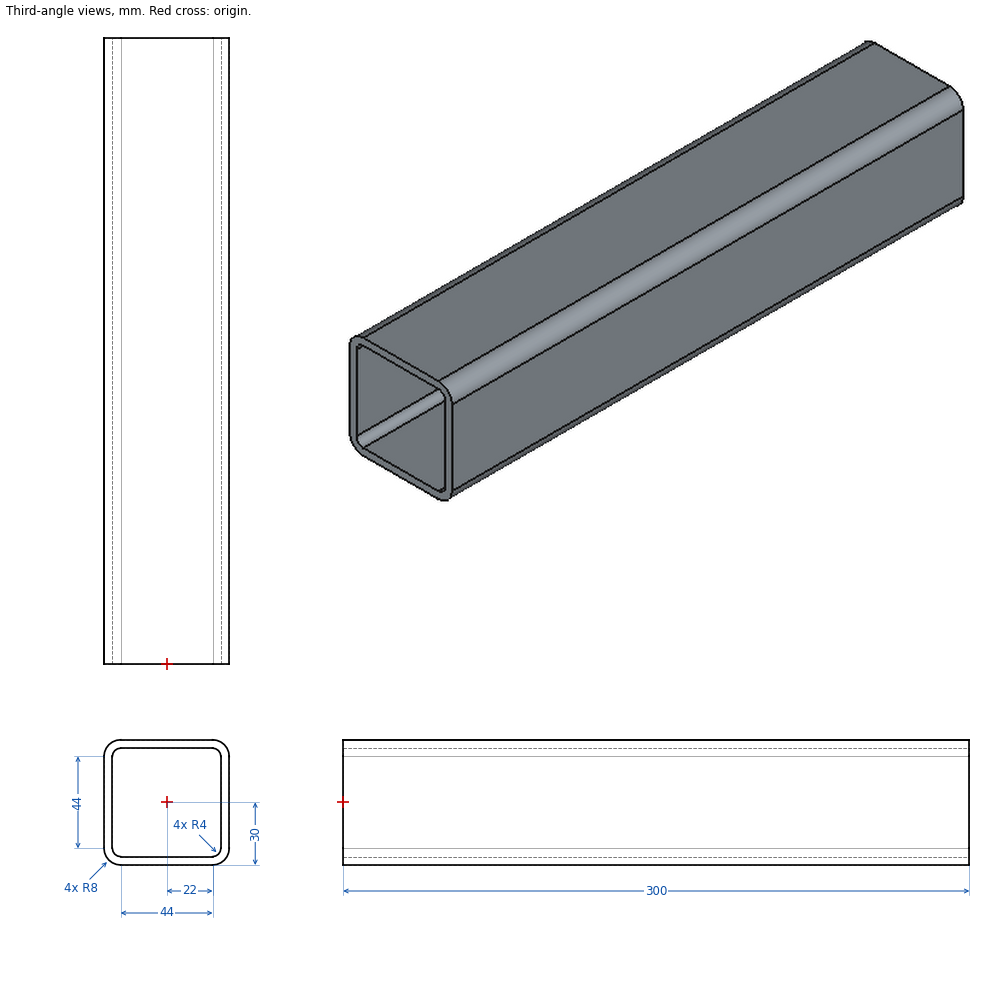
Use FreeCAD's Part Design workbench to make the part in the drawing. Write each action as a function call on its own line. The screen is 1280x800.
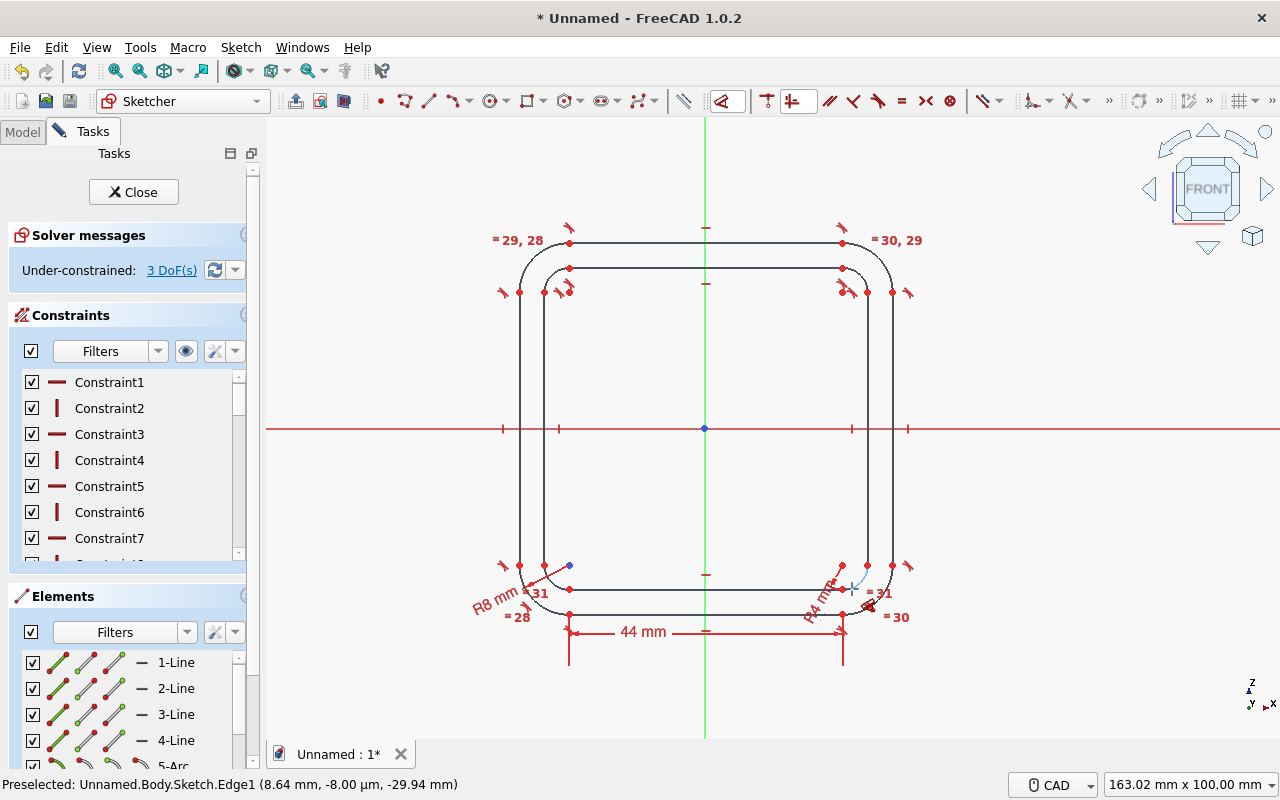
click(520, 483)
click(486, 366)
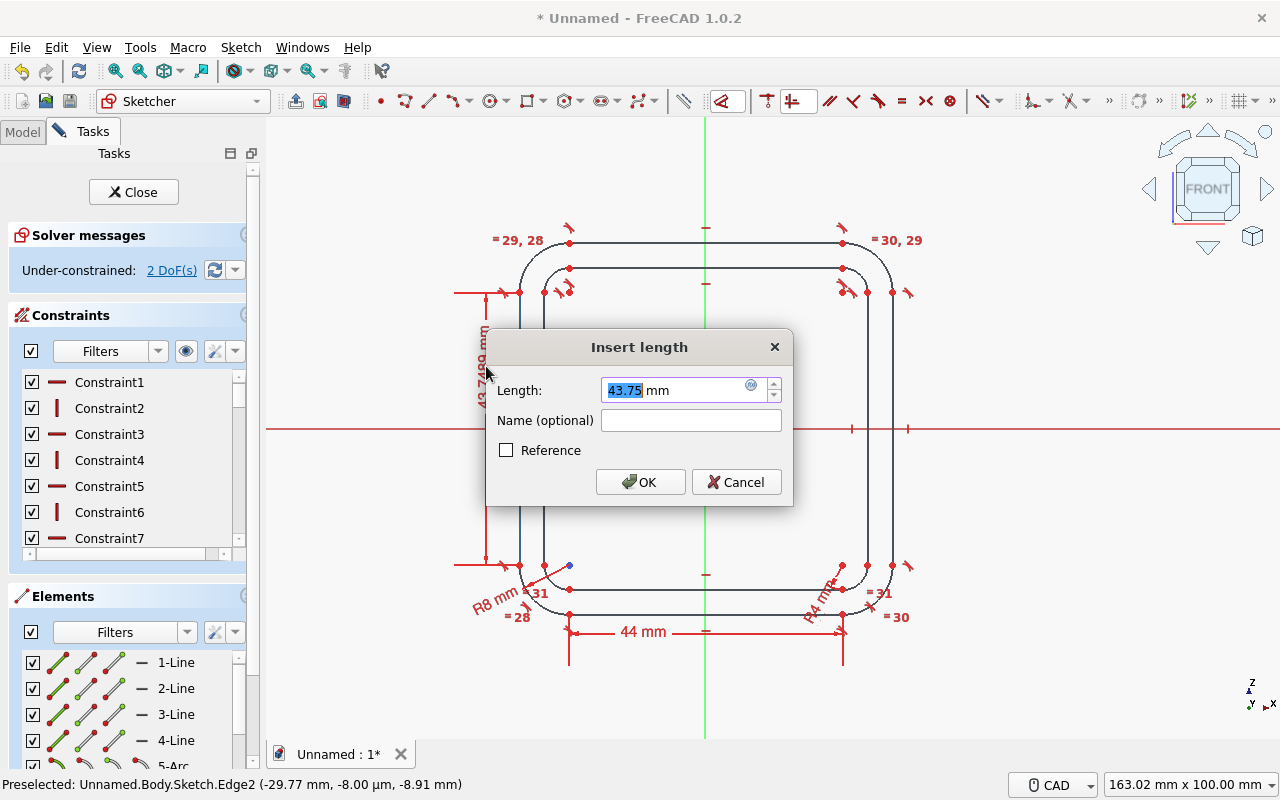
text(44)
key(Return)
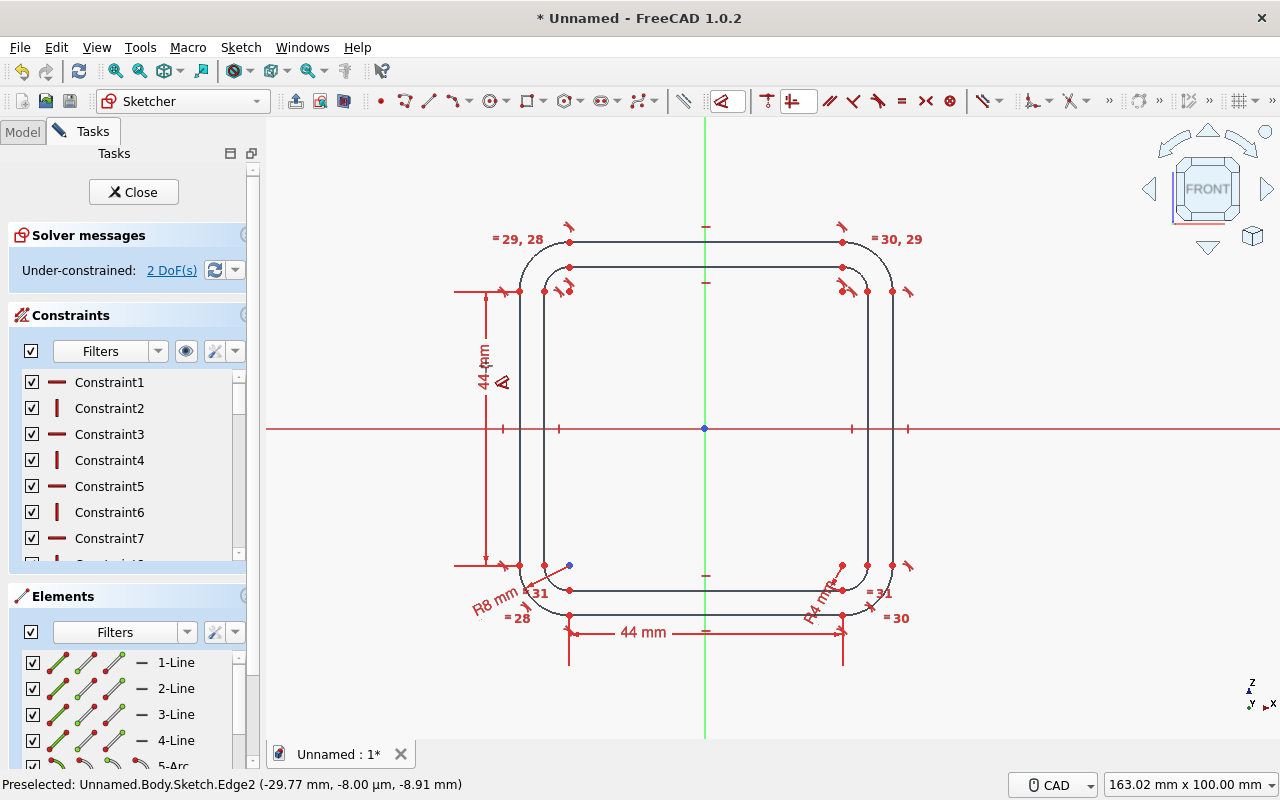
click(843, 615)
click(774, 649)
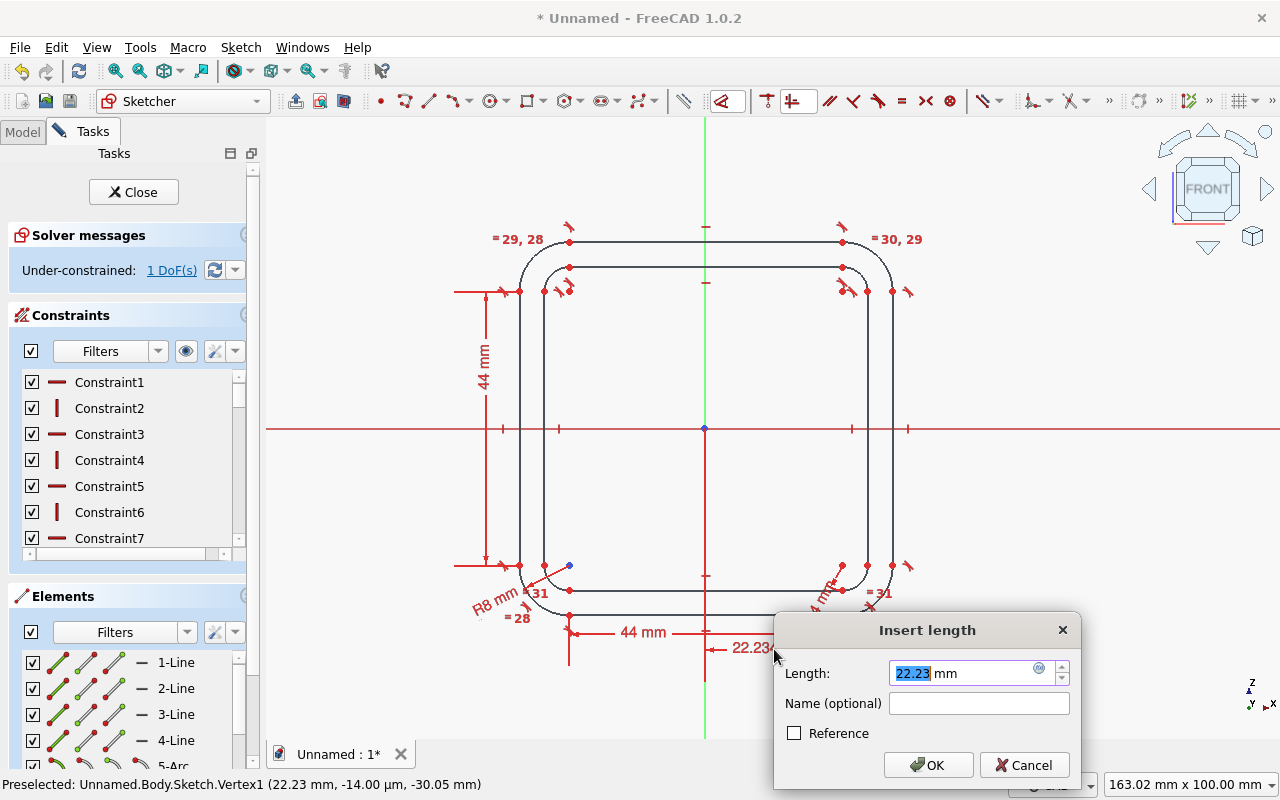
text(22)
key(Return)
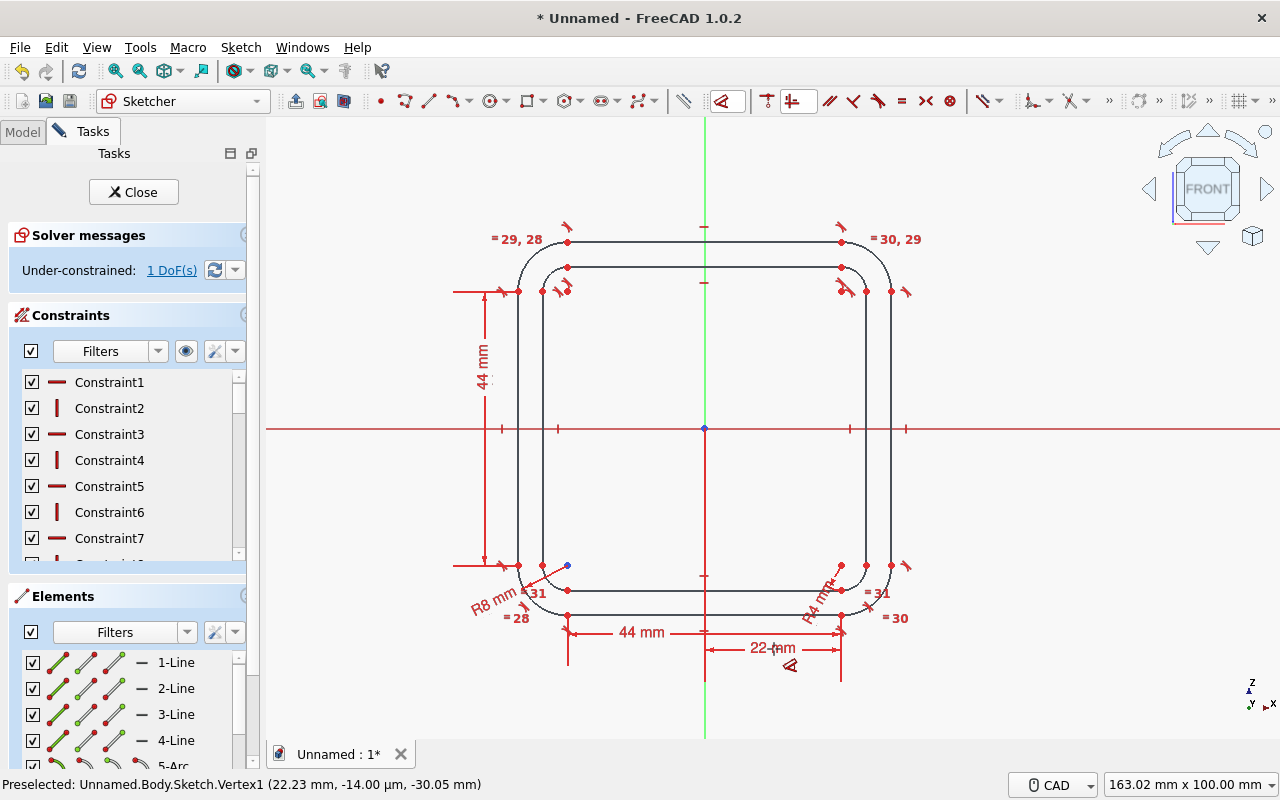
click(841, 615)
click(671, 522)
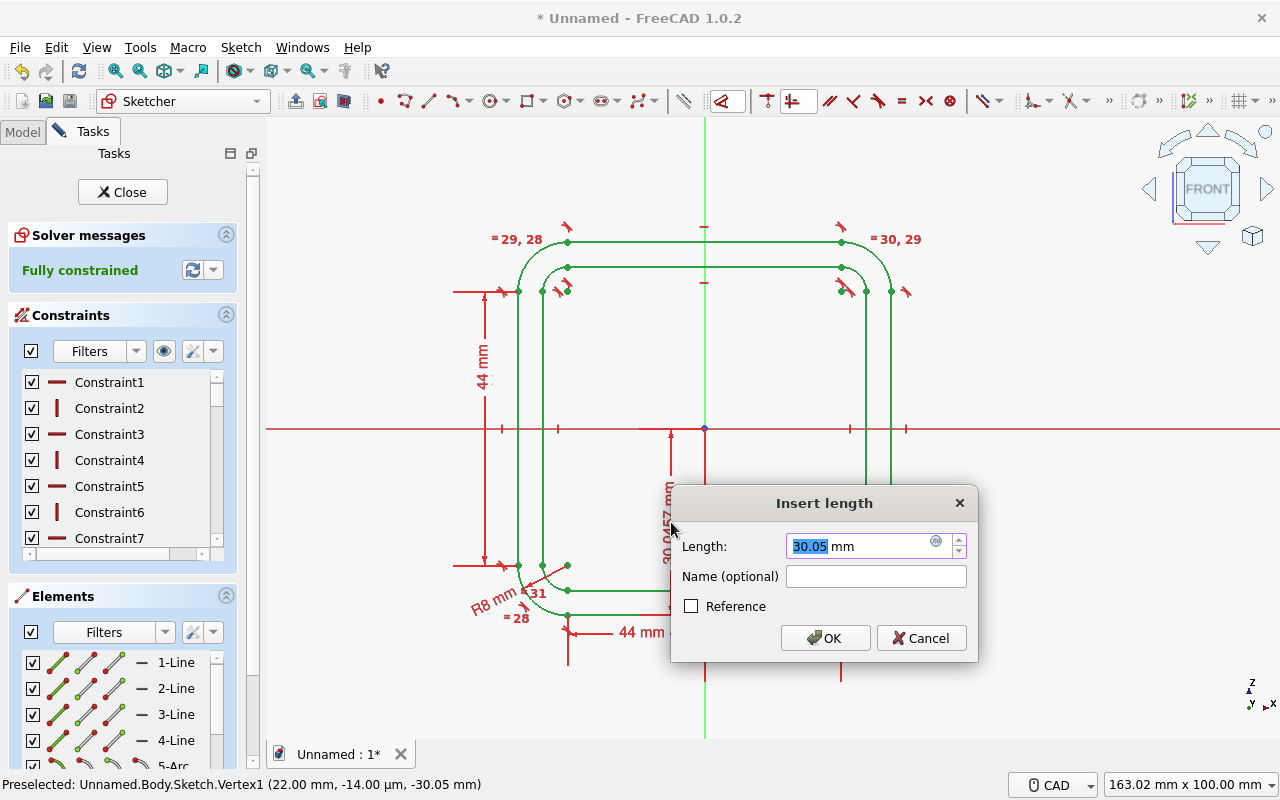
text(30)
key(Return)
key(Escape)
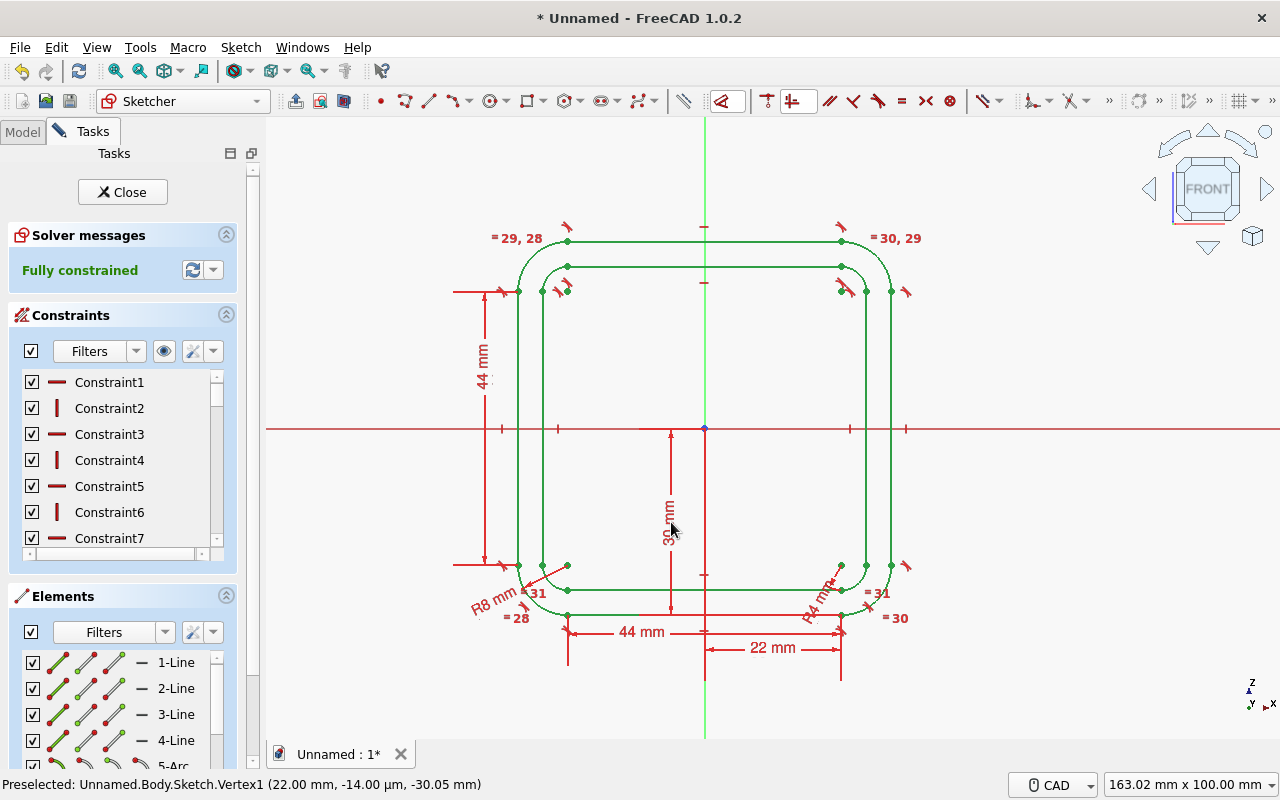
click(123, 192)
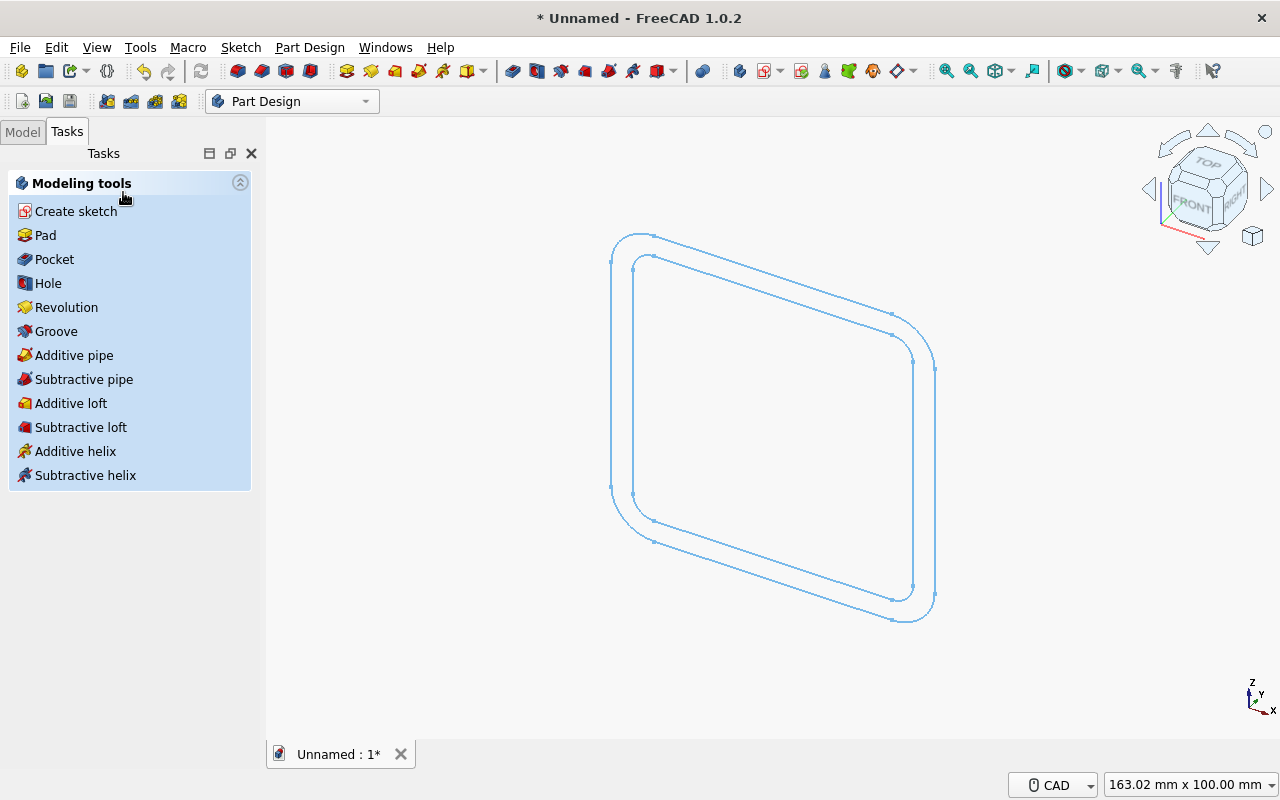
click(348, 72)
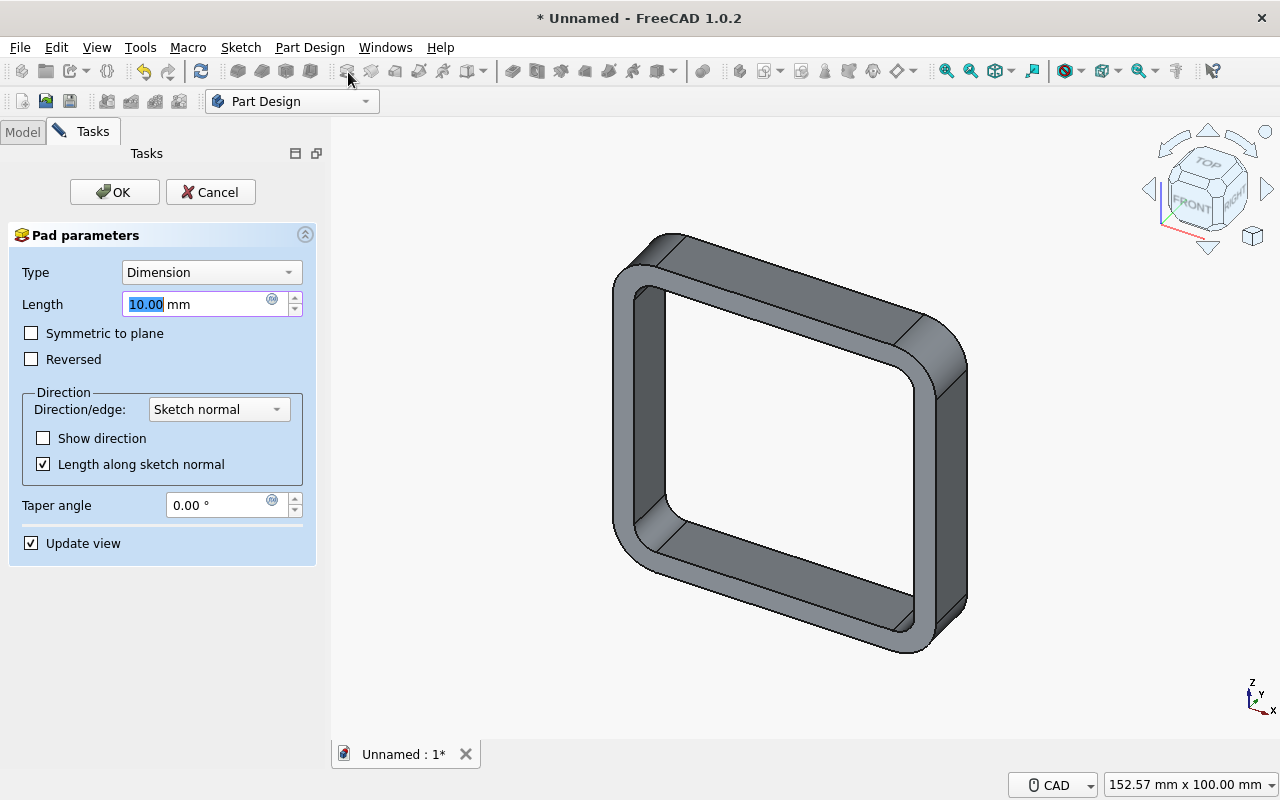
text(300)
key(Tab)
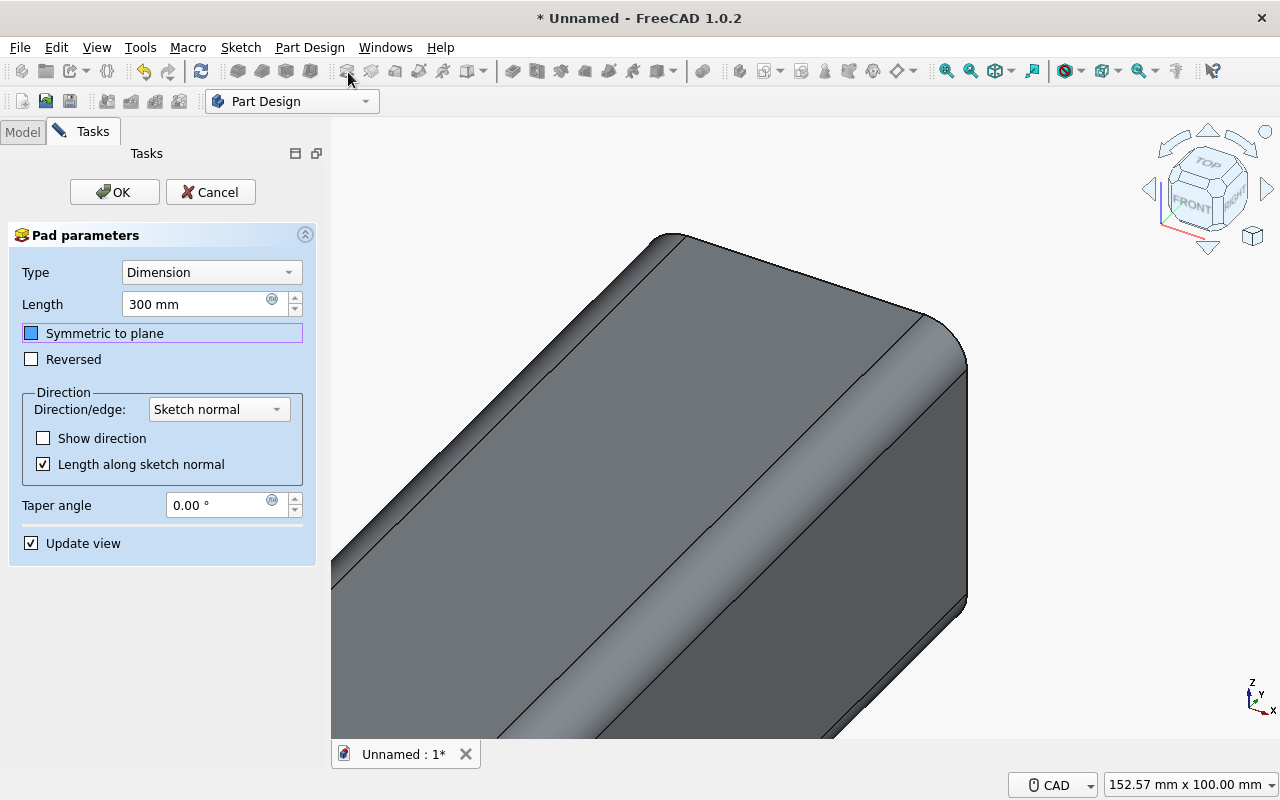
click(30, 359)